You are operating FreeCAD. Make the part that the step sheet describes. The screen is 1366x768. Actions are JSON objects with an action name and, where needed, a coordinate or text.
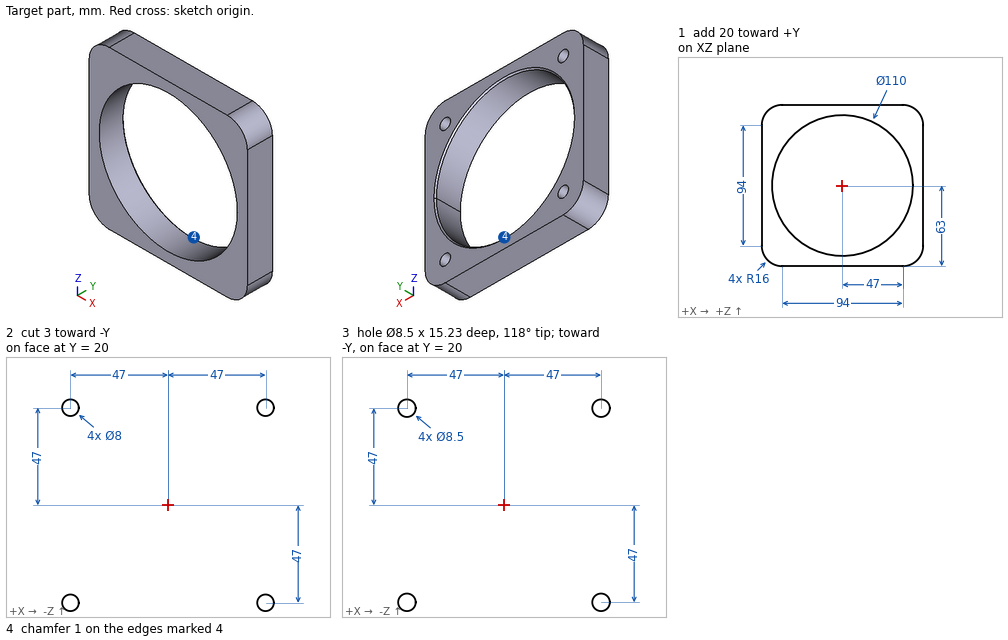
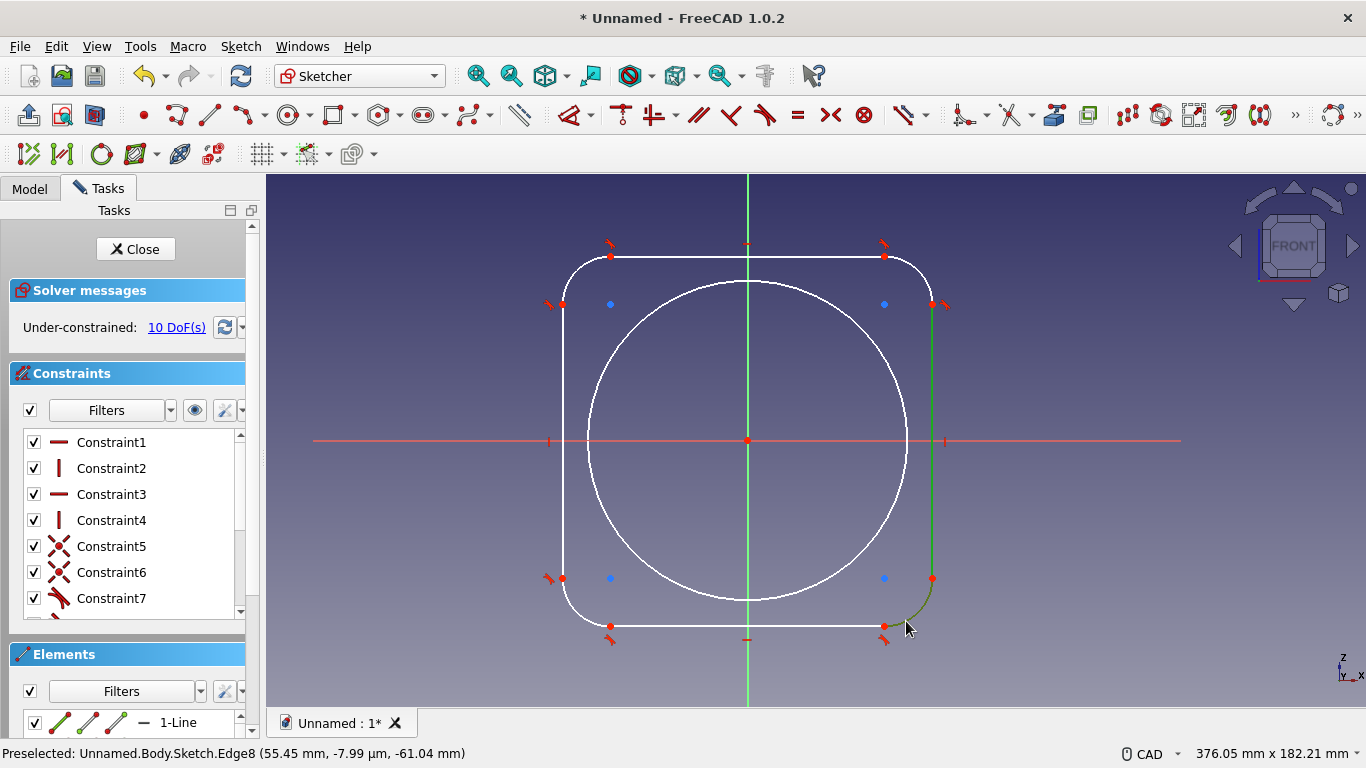
{"action": "left_click", "coordinate": [765, 116]}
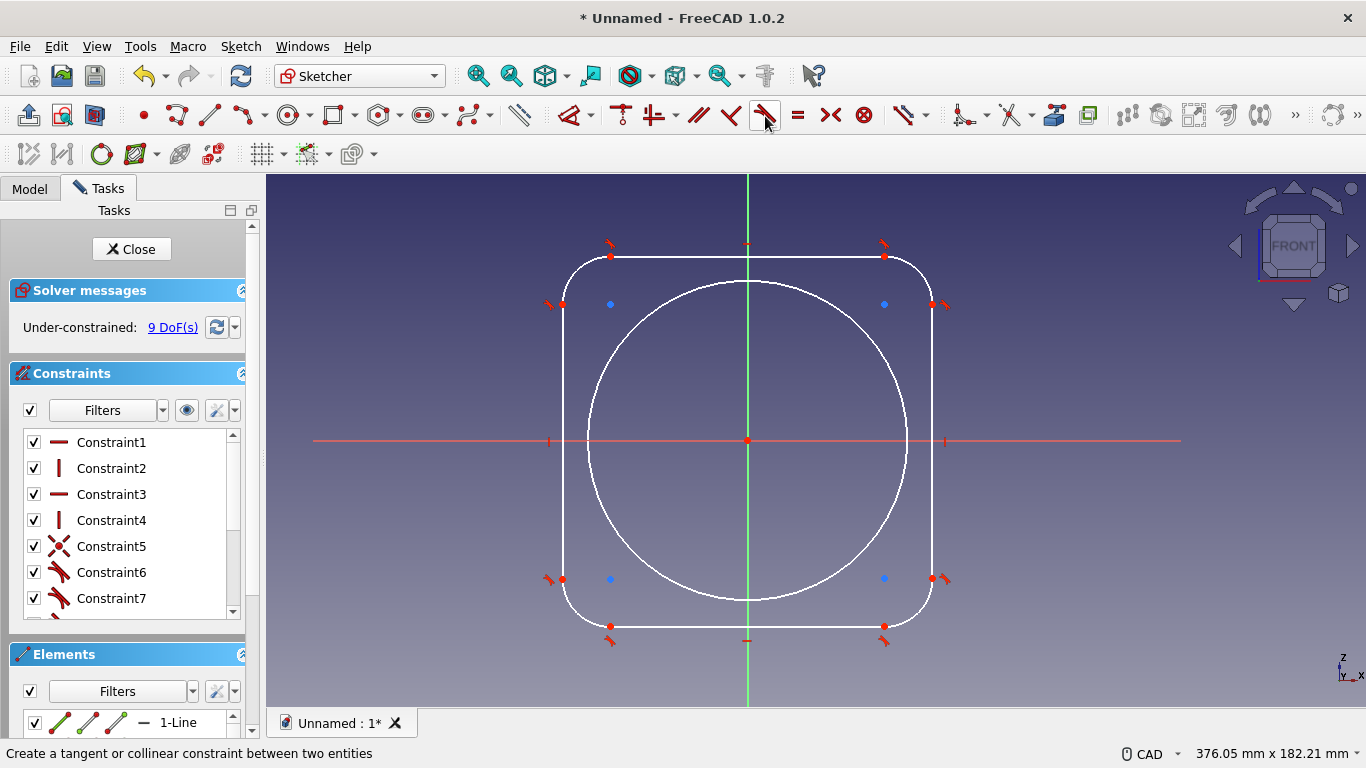
{"action": "left_click", "coordinate": [568, 601]}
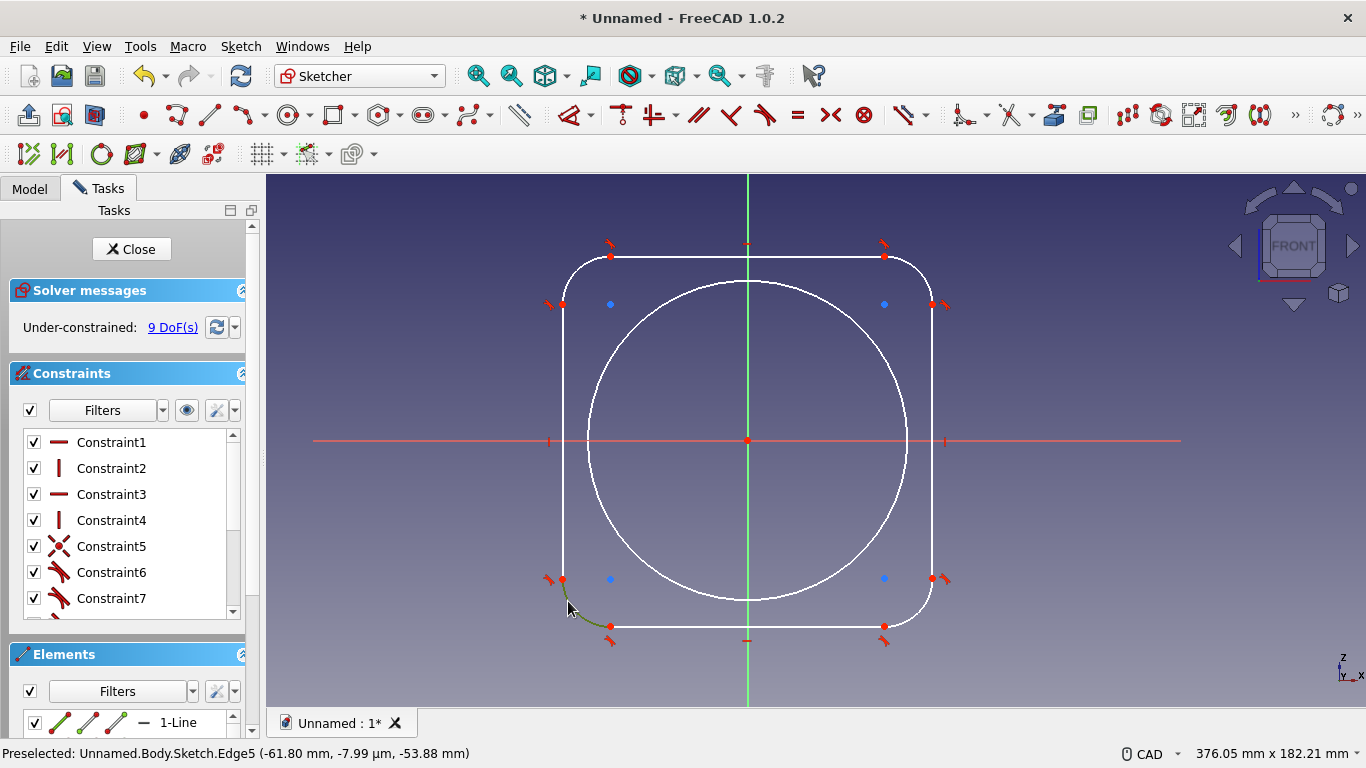
{"action": "left_click", "coordinate": [589, 262]}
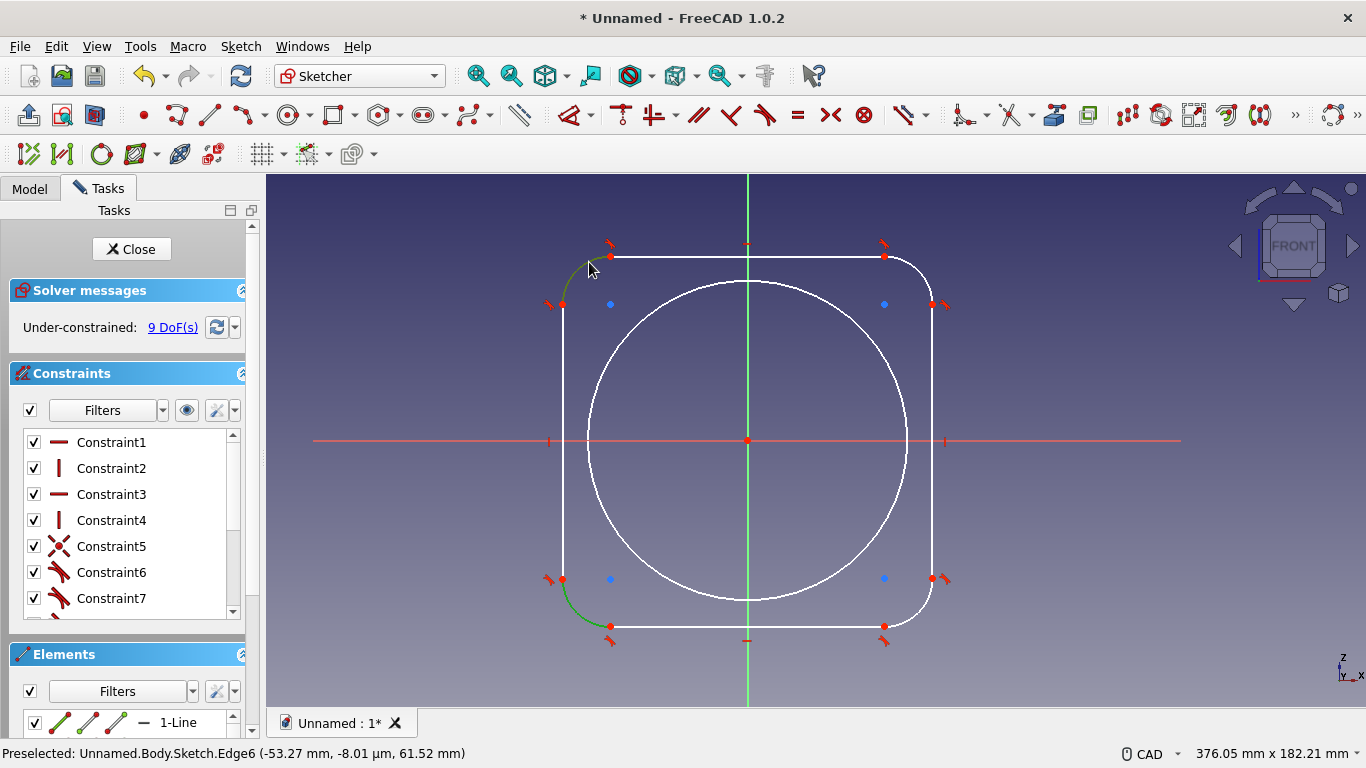
{"action": "left_click", "coordinate": [927, 283]}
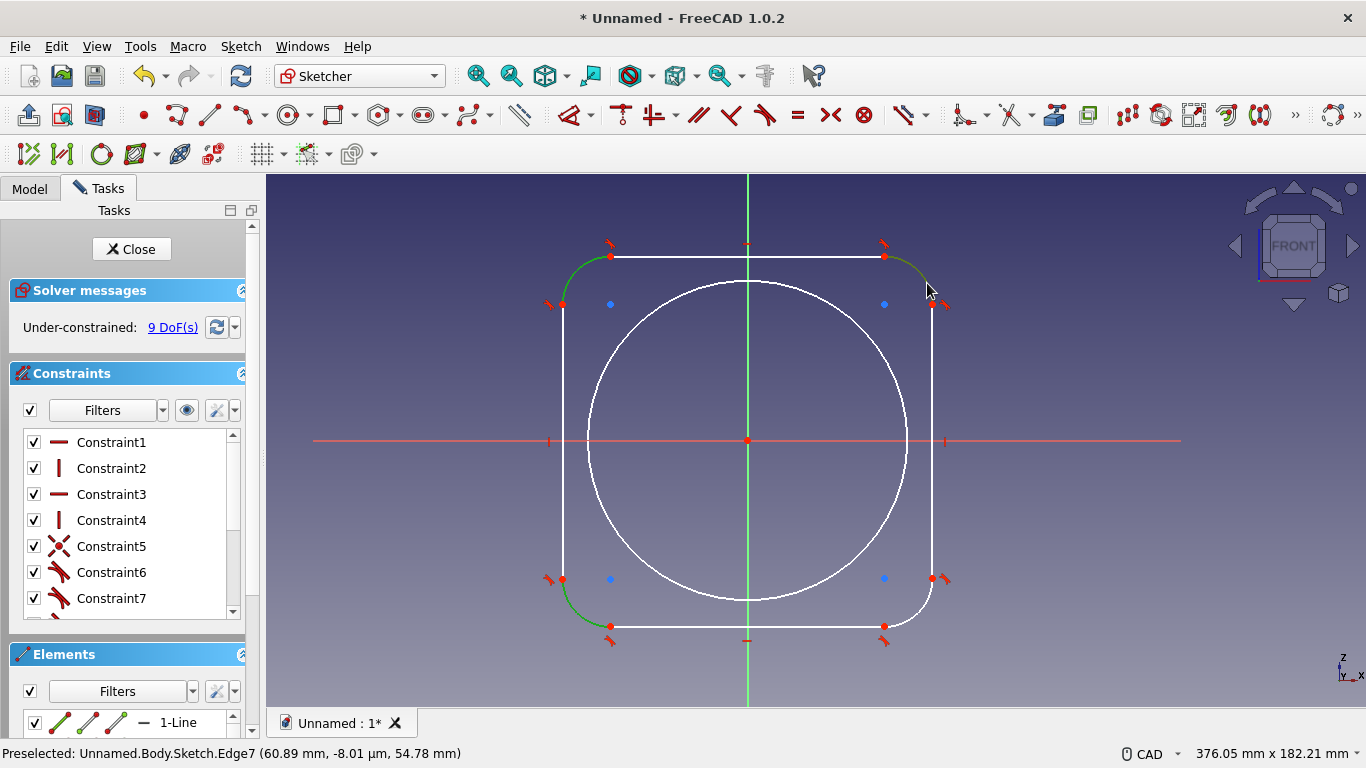
{"action": "left_click", "coordinate": [906, 622]}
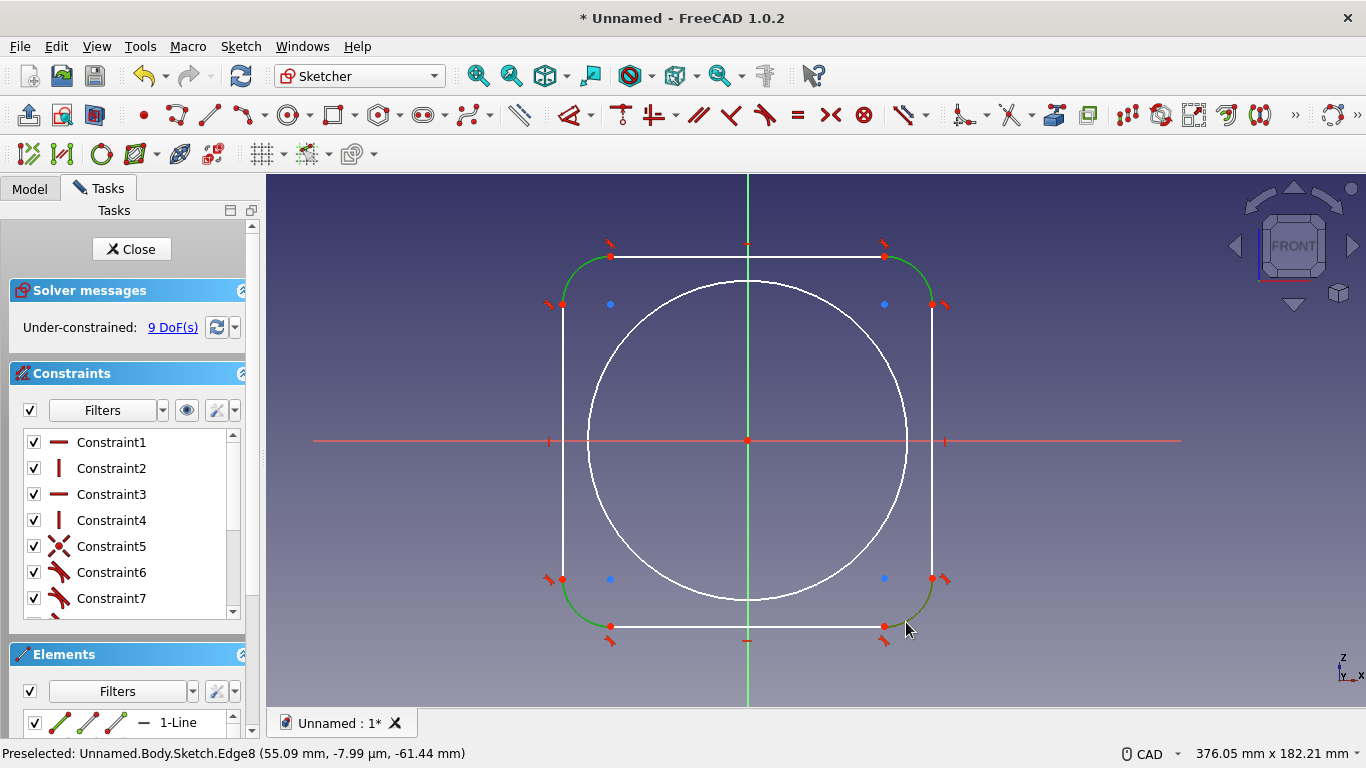
{"action": "left_click", "coordinate": [798, 116]}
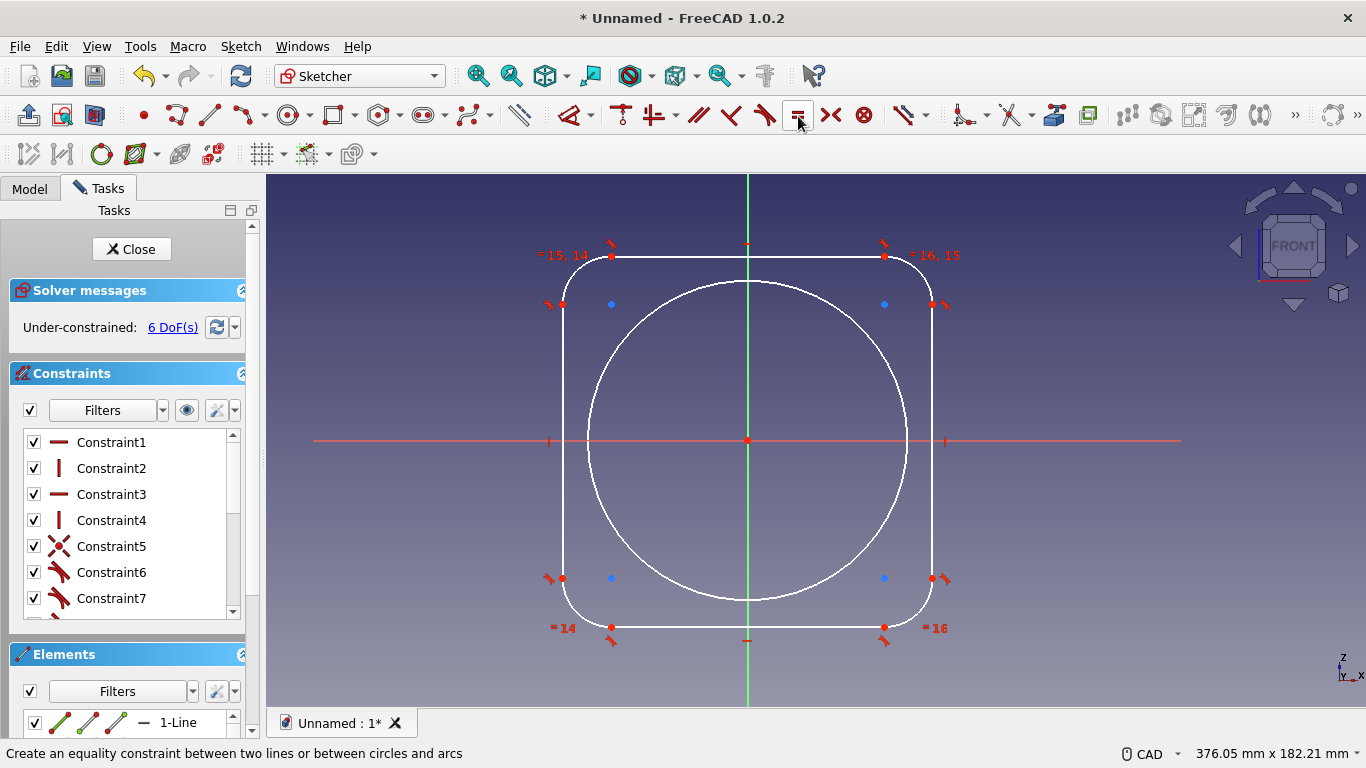
{"action": "left_click", "coordinate": [568, 601]}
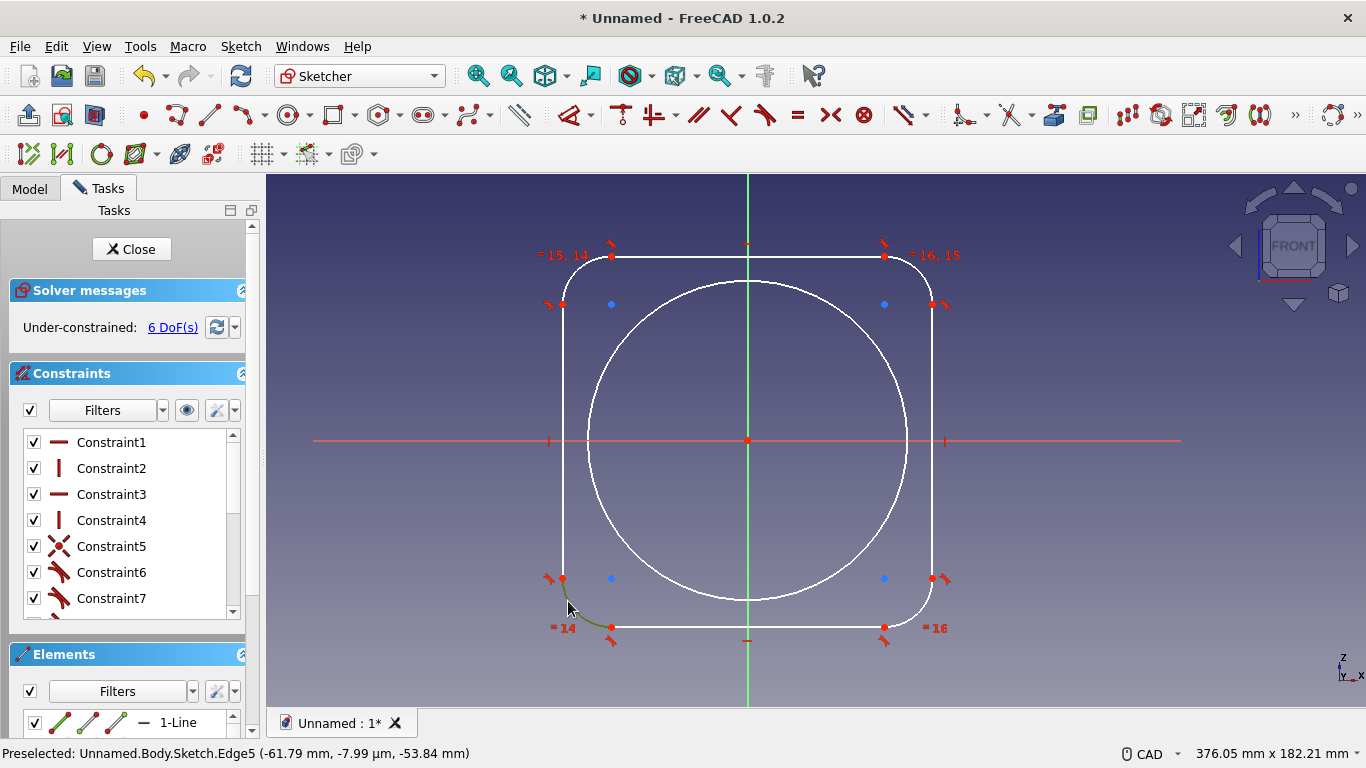
{"action": "left_click", "coordinate": [590, 116]}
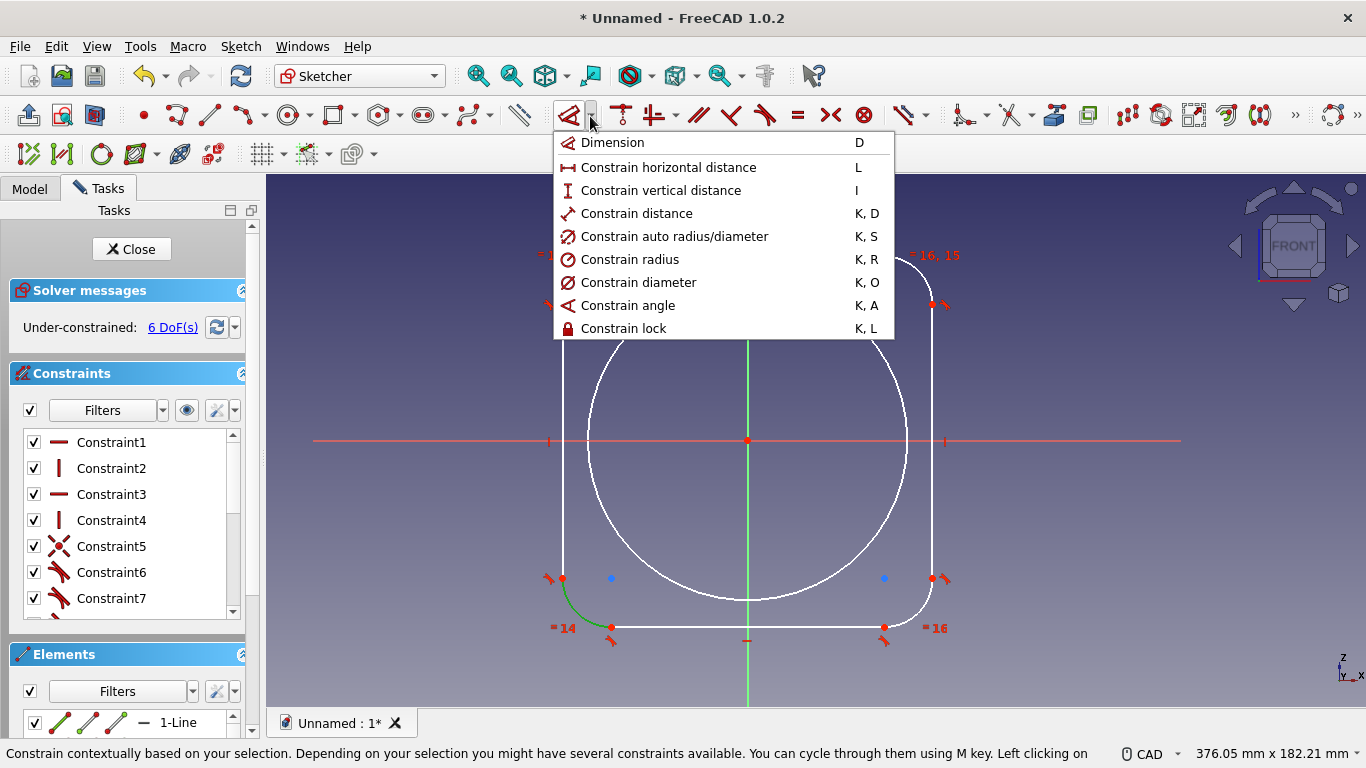
{"action": "left_click", "coordinate": [724, 260]}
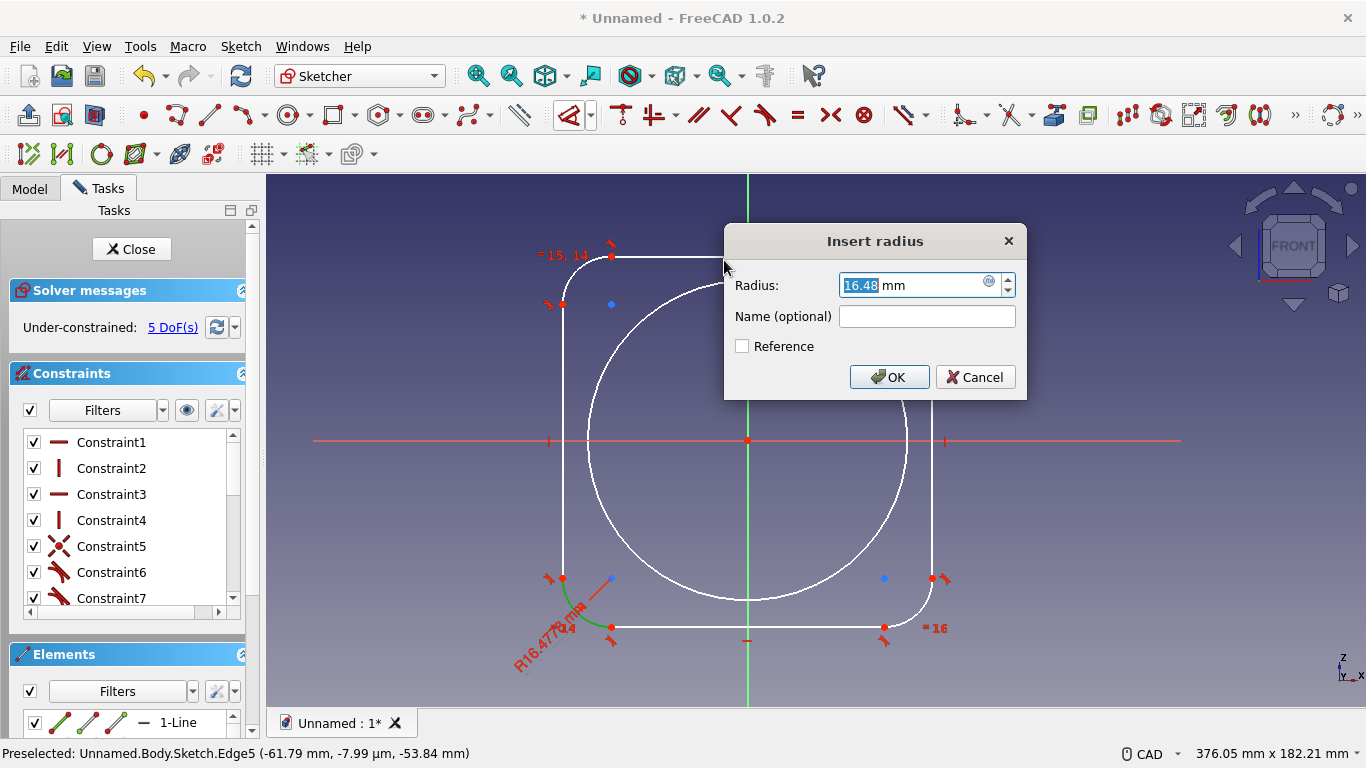
{"action": "type", "text": "16"}
{"action": "key", "text": "Return"}